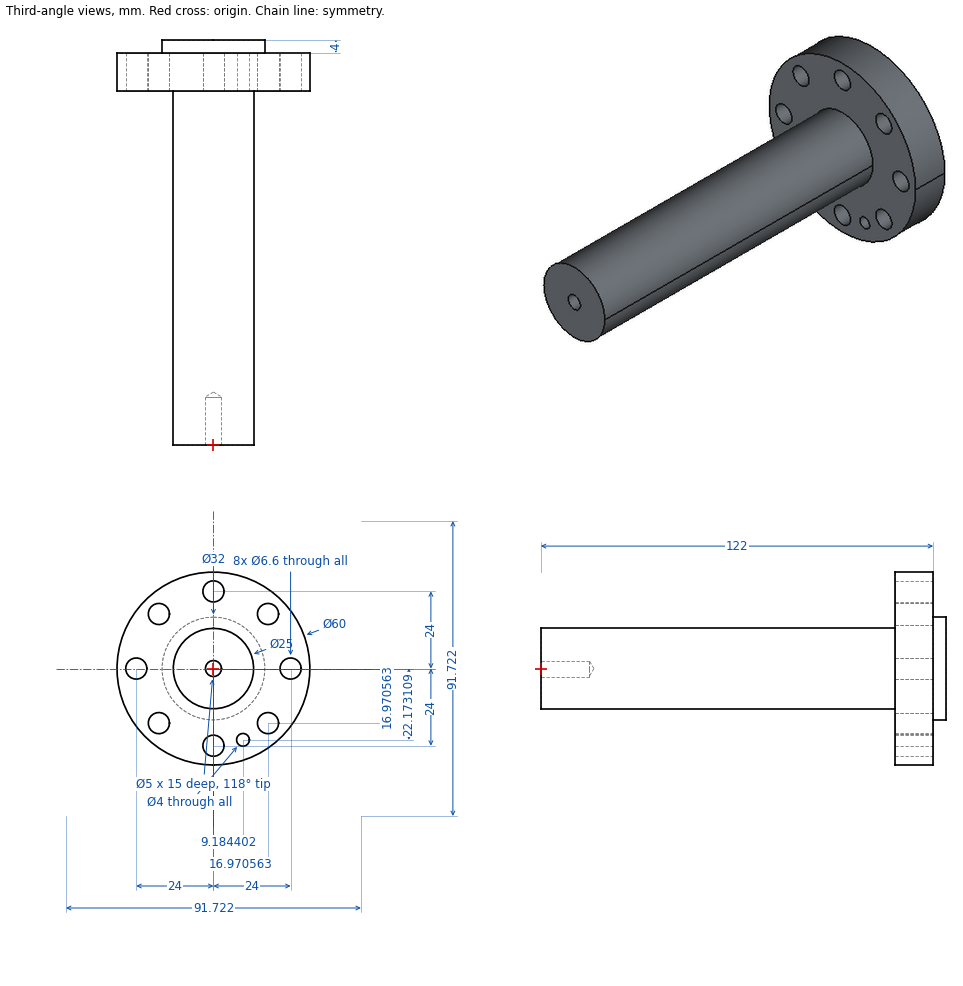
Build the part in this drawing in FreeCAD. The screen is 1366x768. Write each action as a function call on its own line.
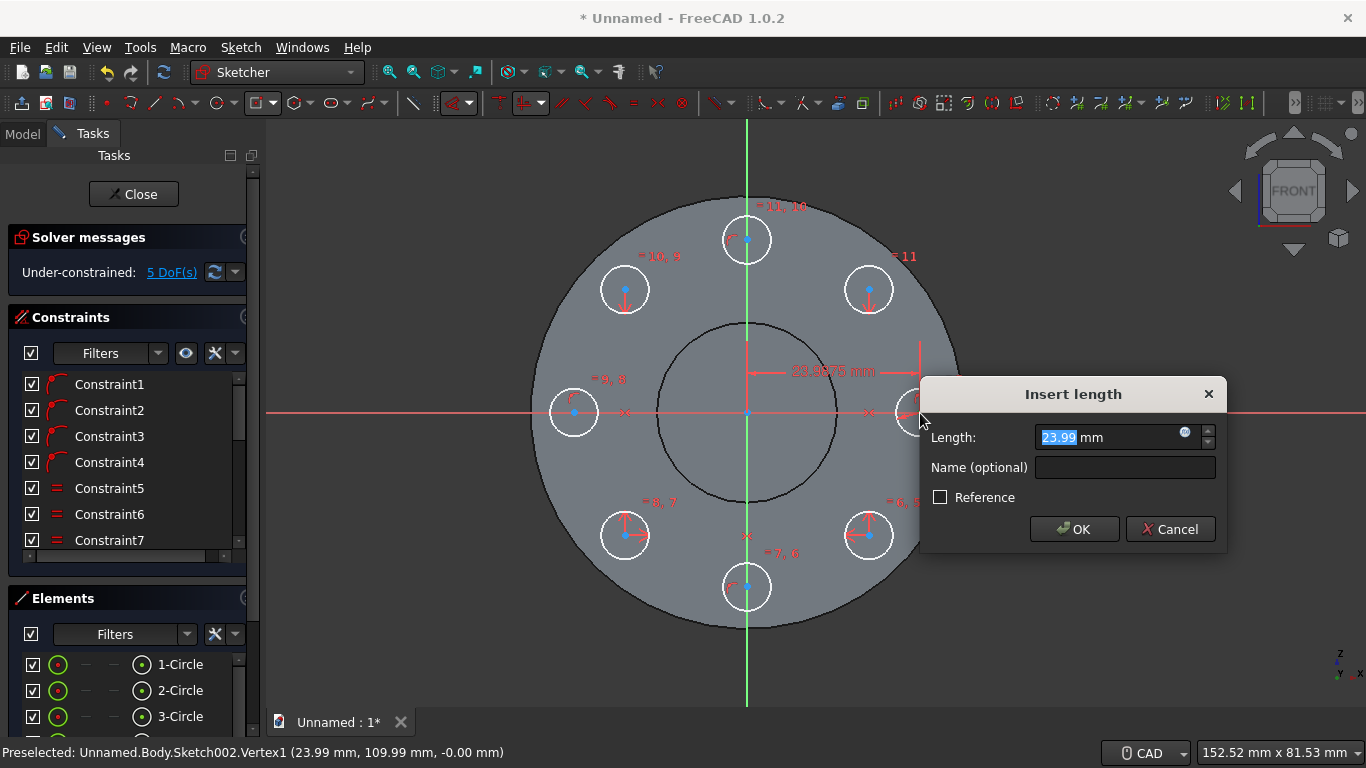
text(24)
key(Return)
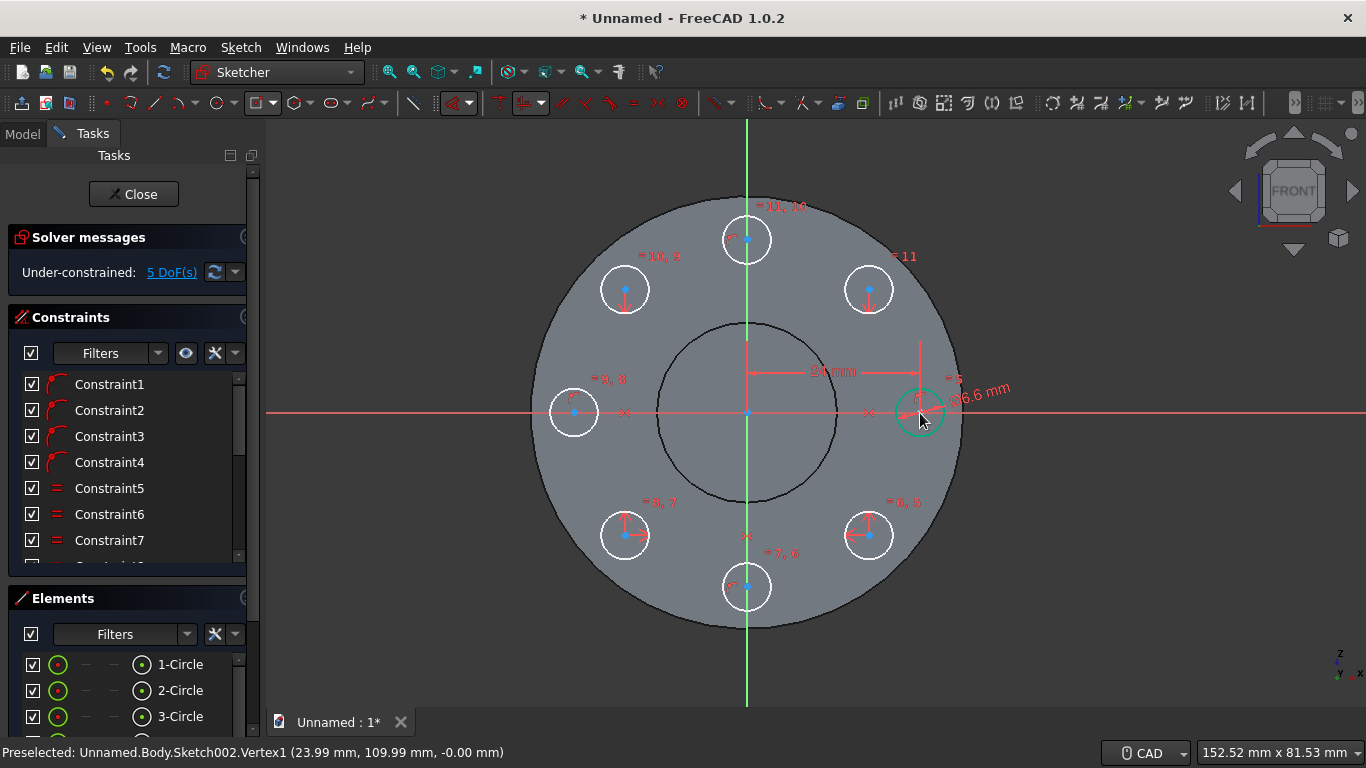
click(747, 587)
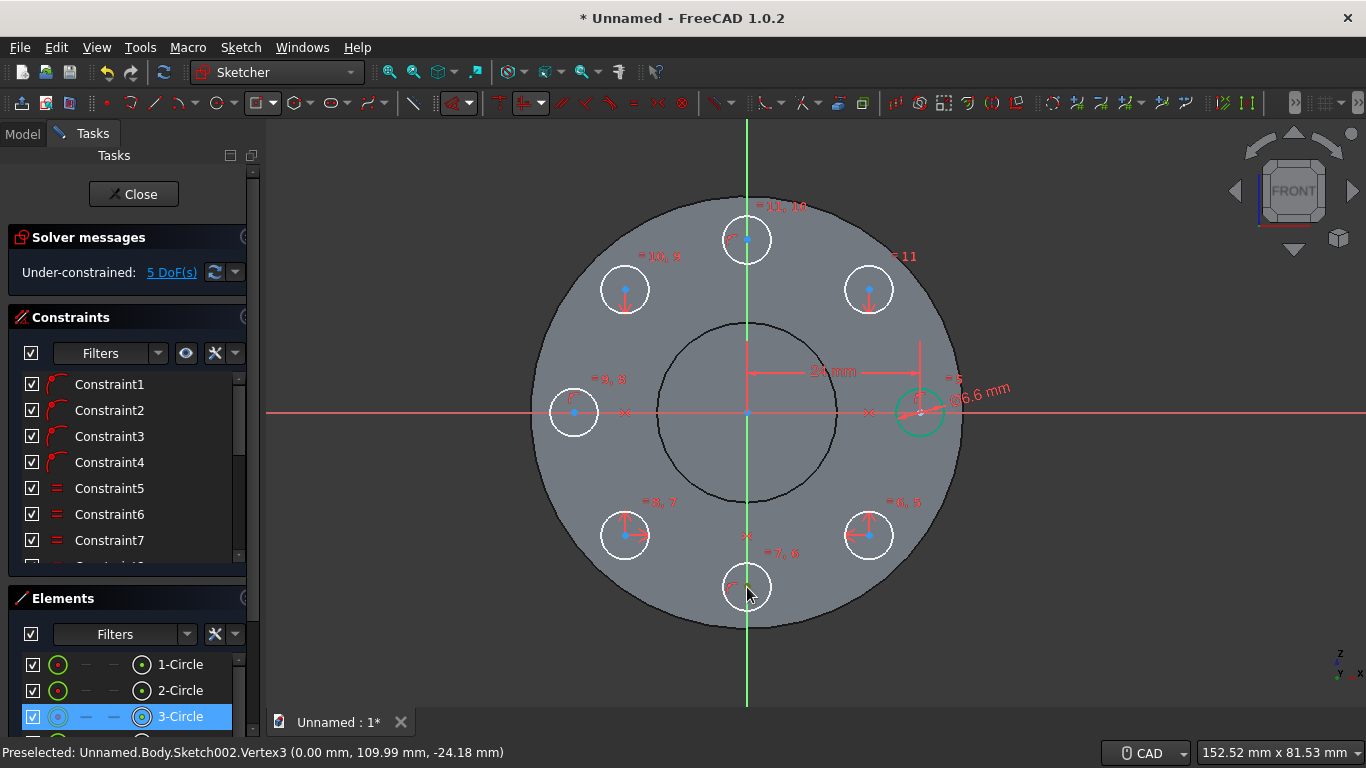
key(i)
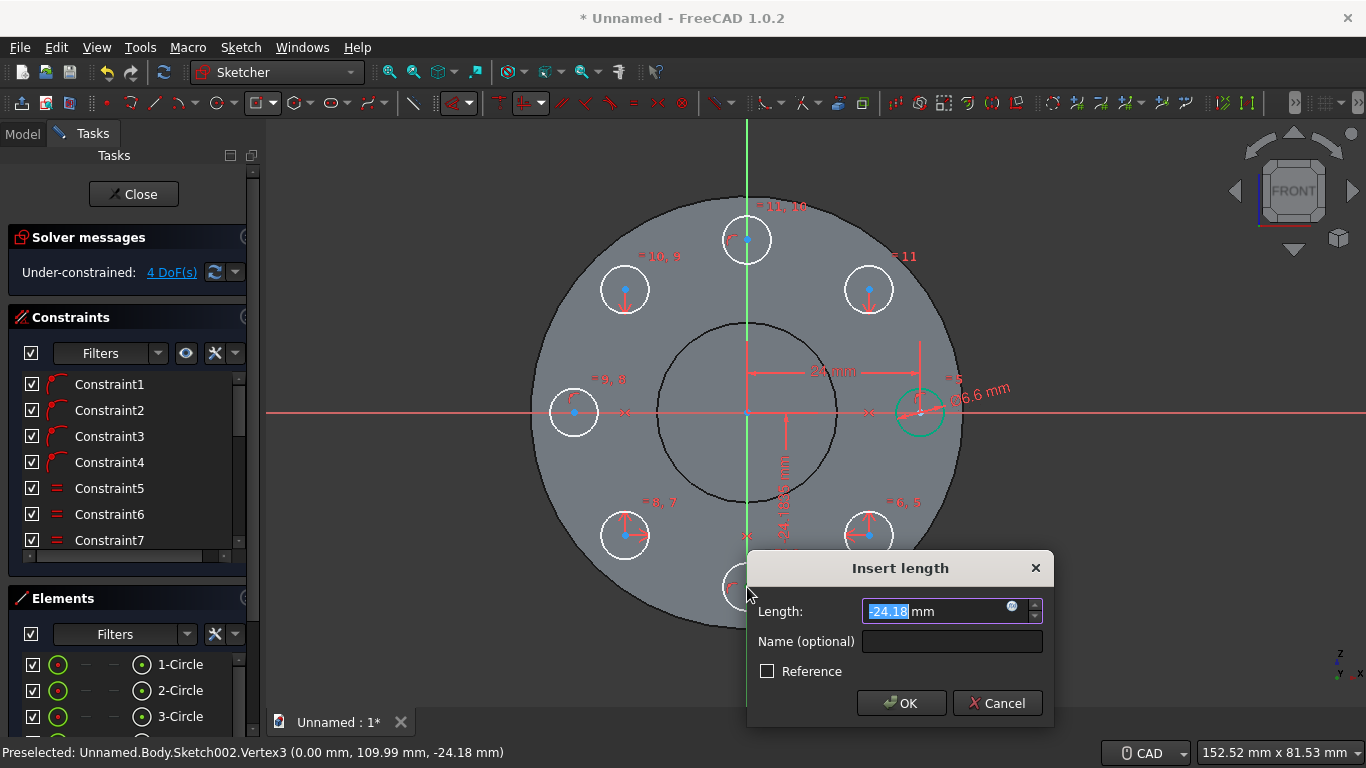
text(-24)
key(Return)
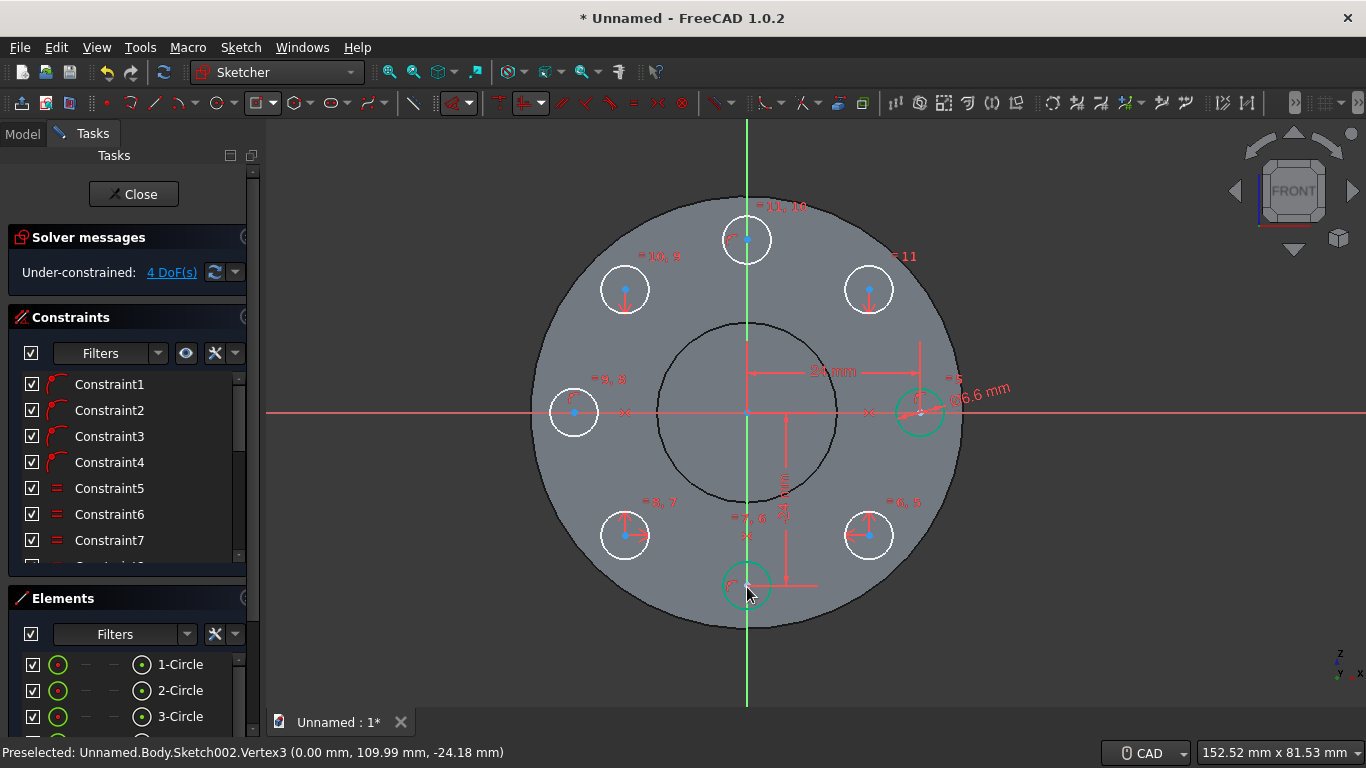
click(574, 413)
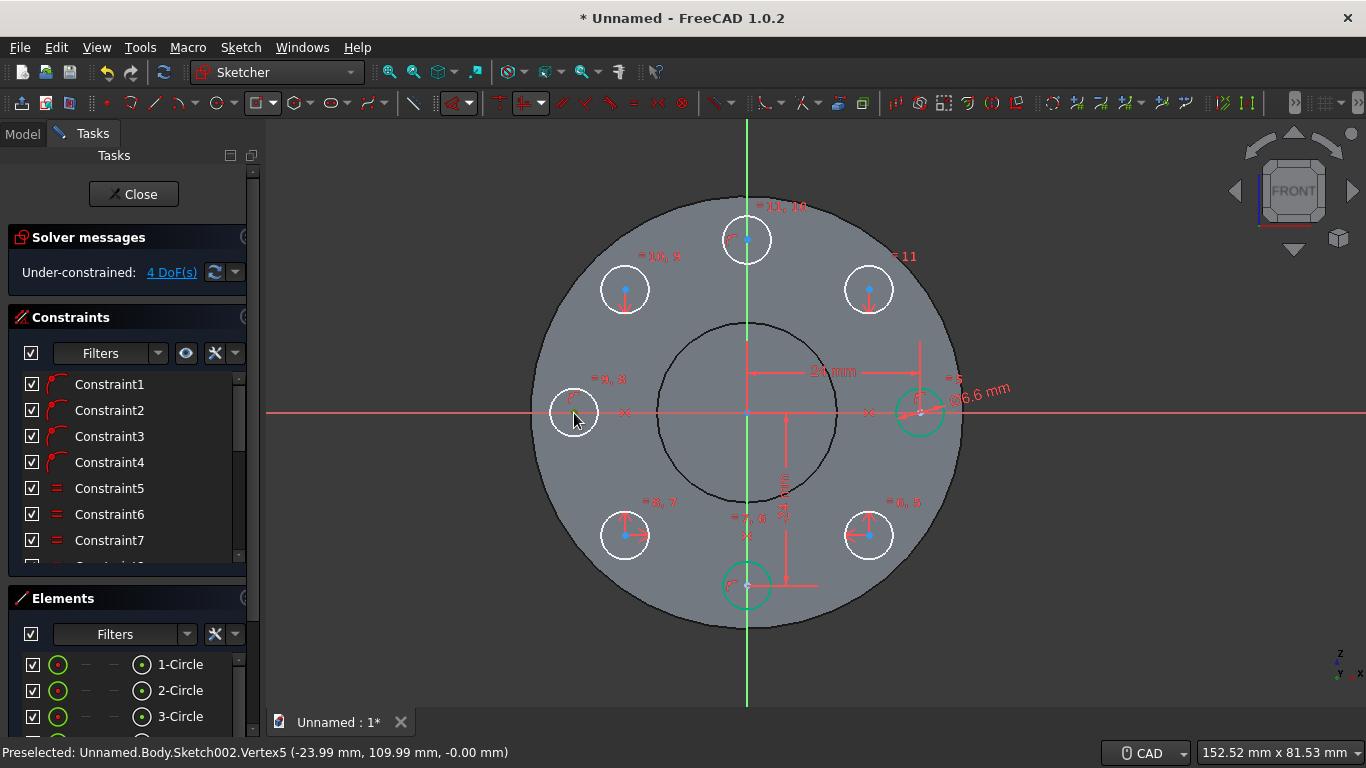
click(472, 104)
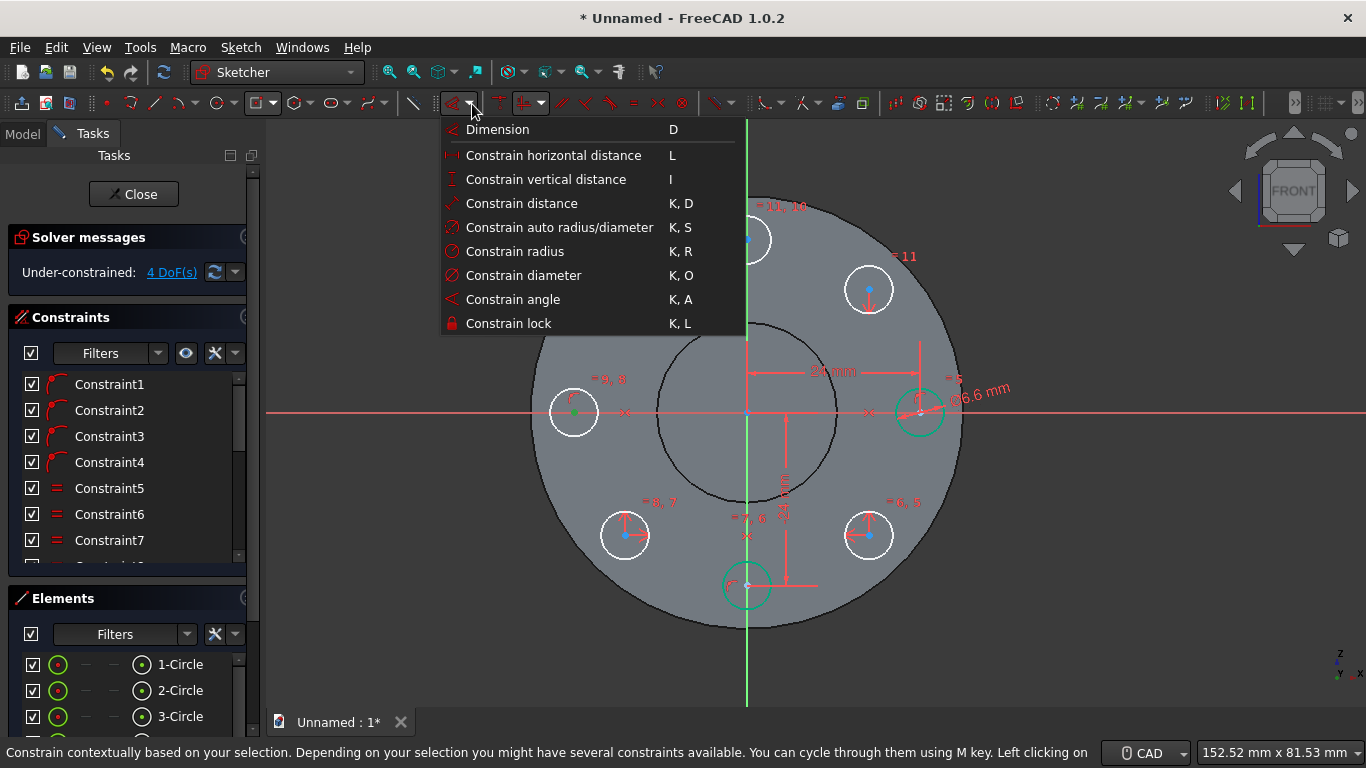
click(593, 155)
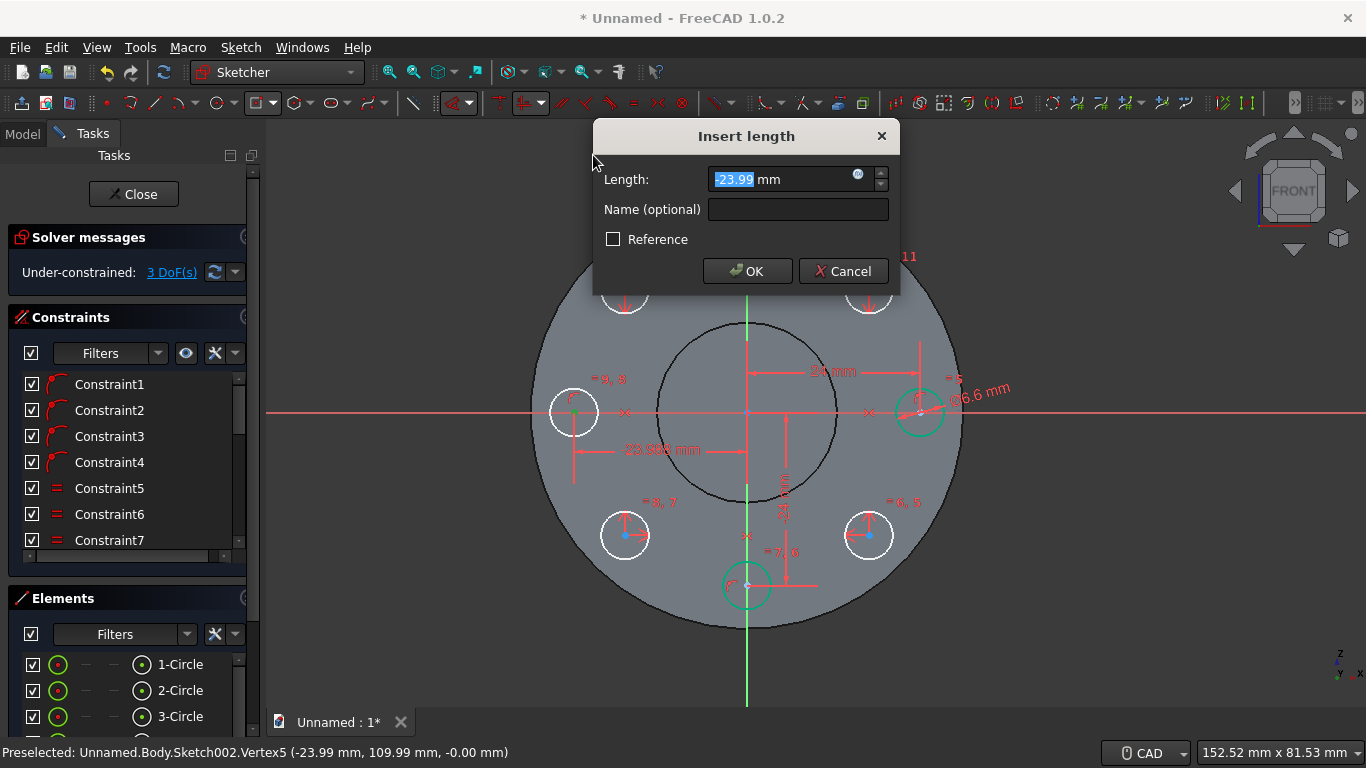
text(-24)
key(Return)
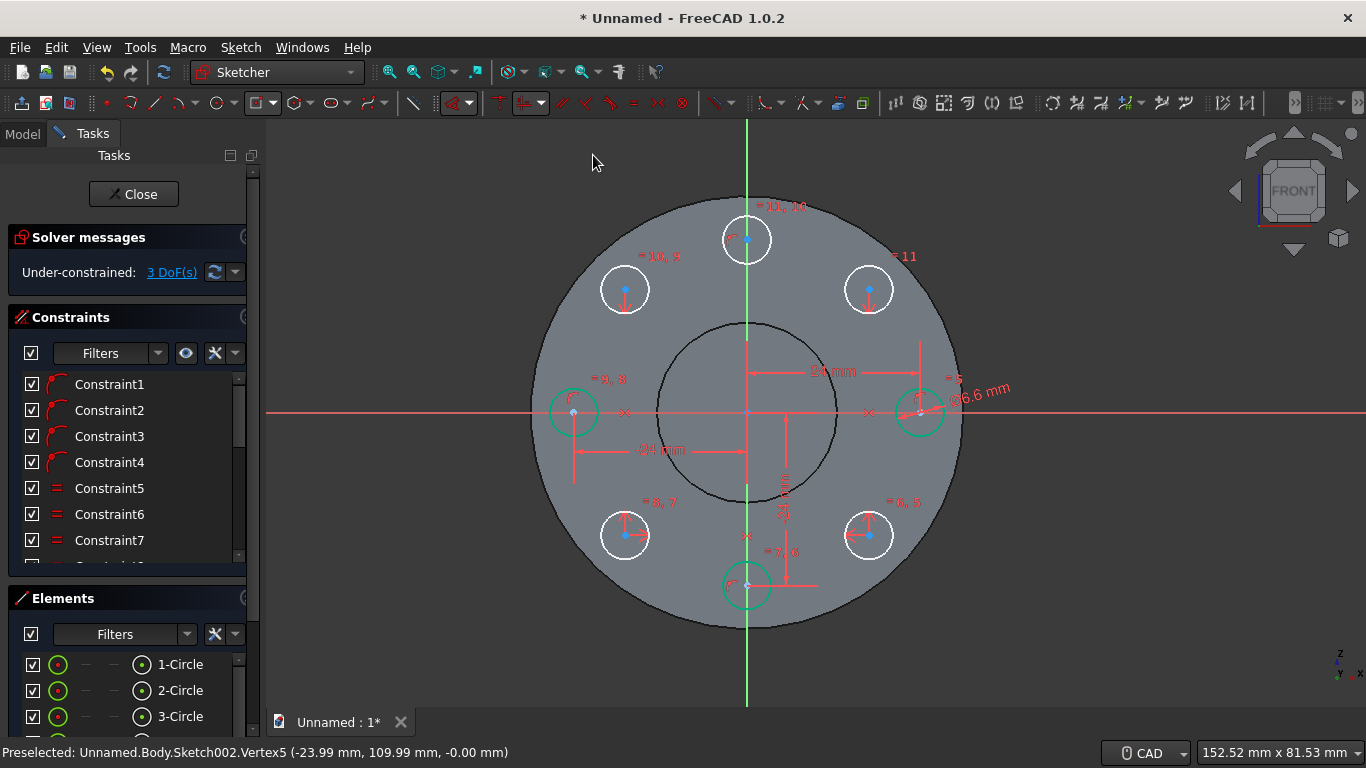
click(747, 240)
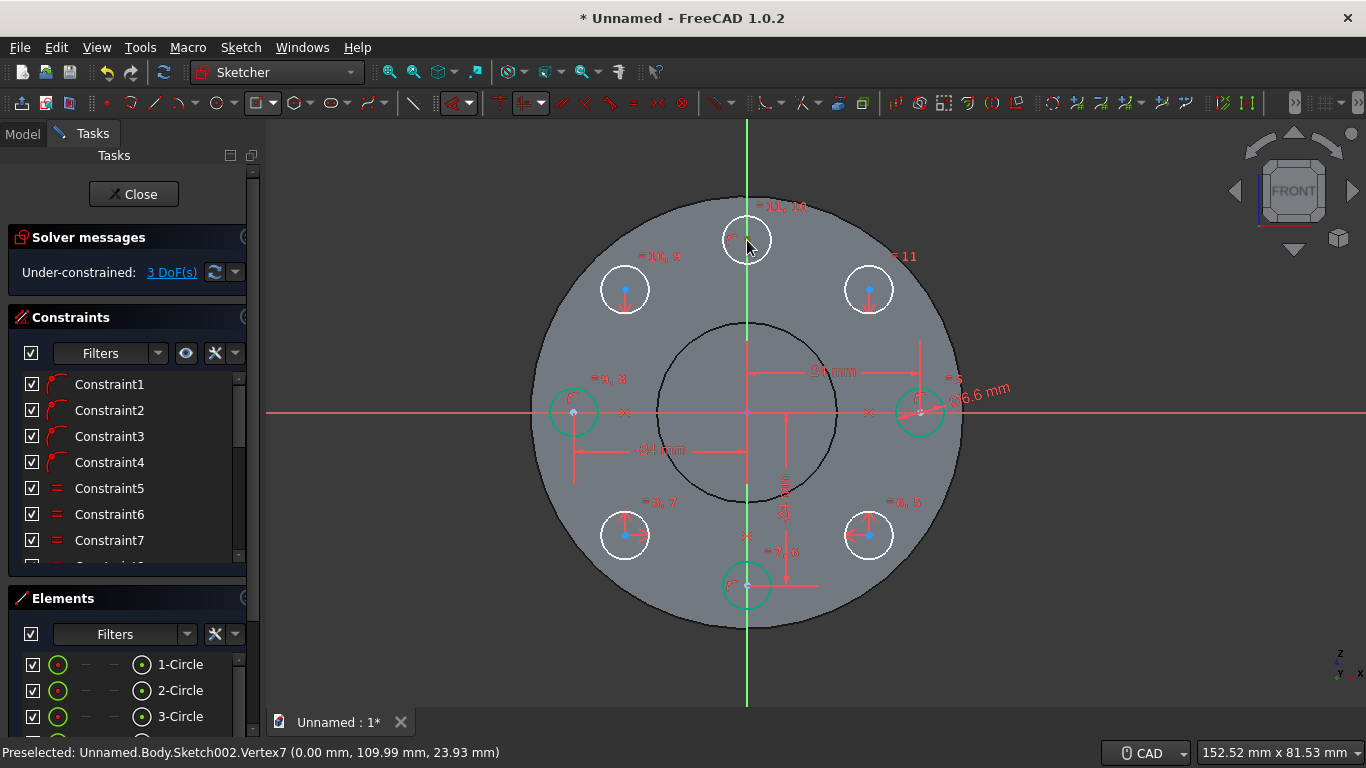
click(472, 104)